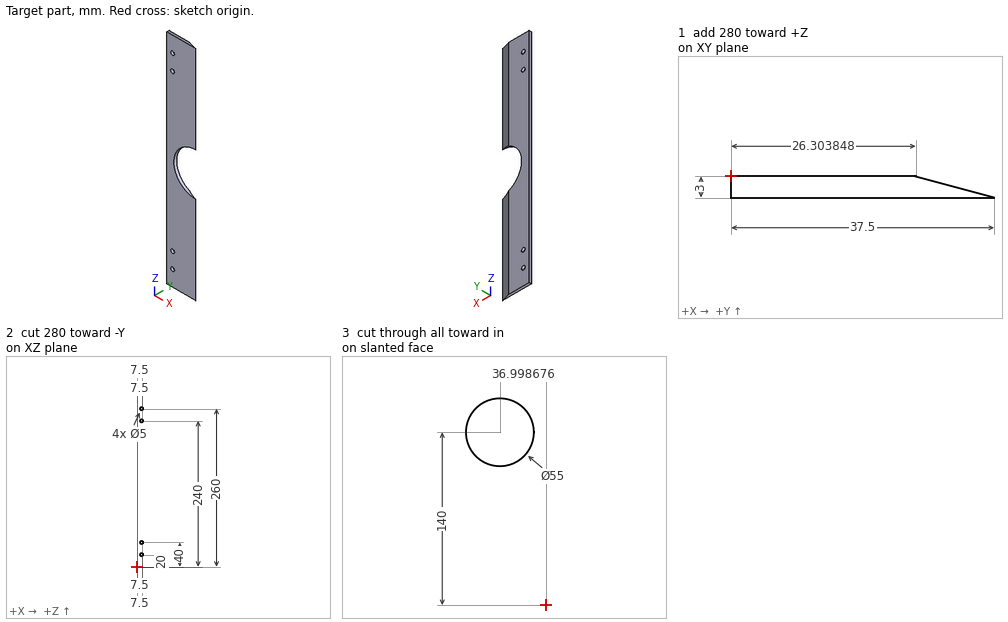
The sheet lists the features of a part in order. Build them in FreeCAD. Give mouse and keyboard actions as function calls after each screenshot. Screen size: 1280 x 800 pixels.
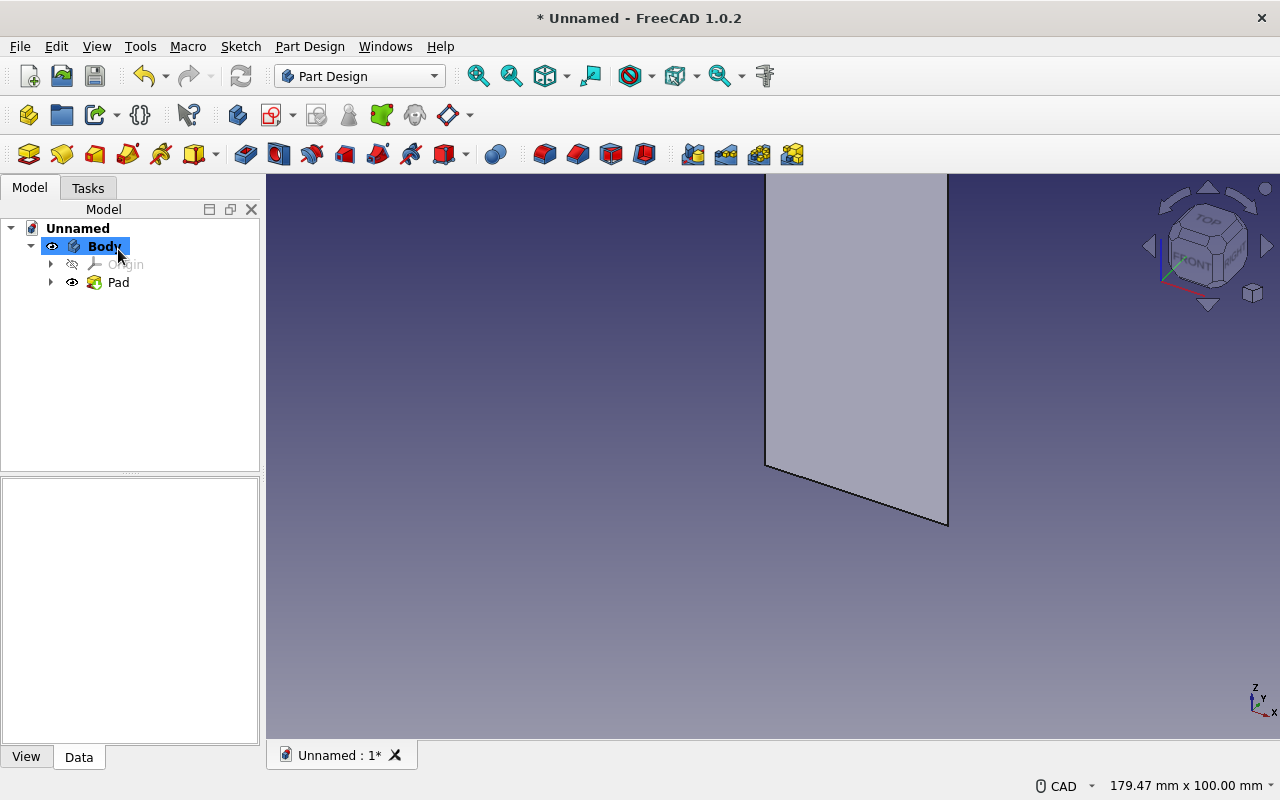
click(479, 76)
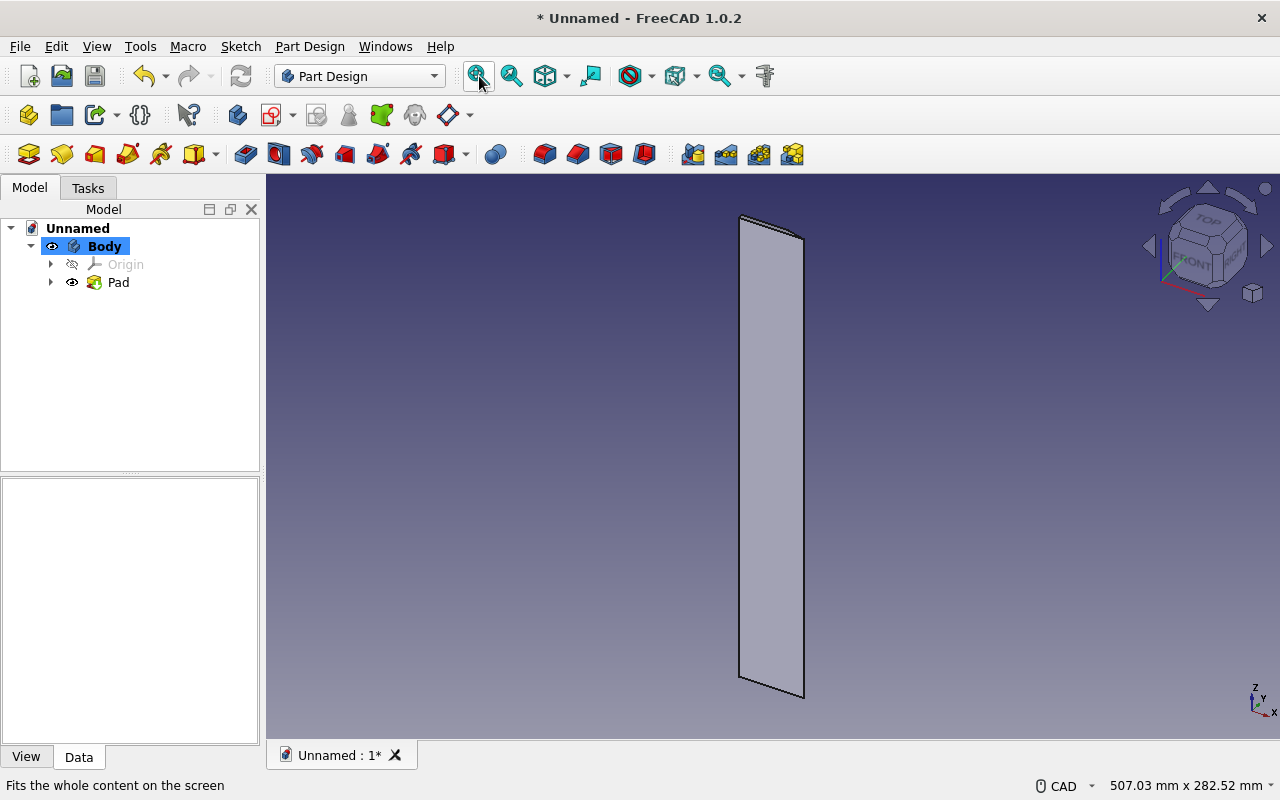
click(270, 116)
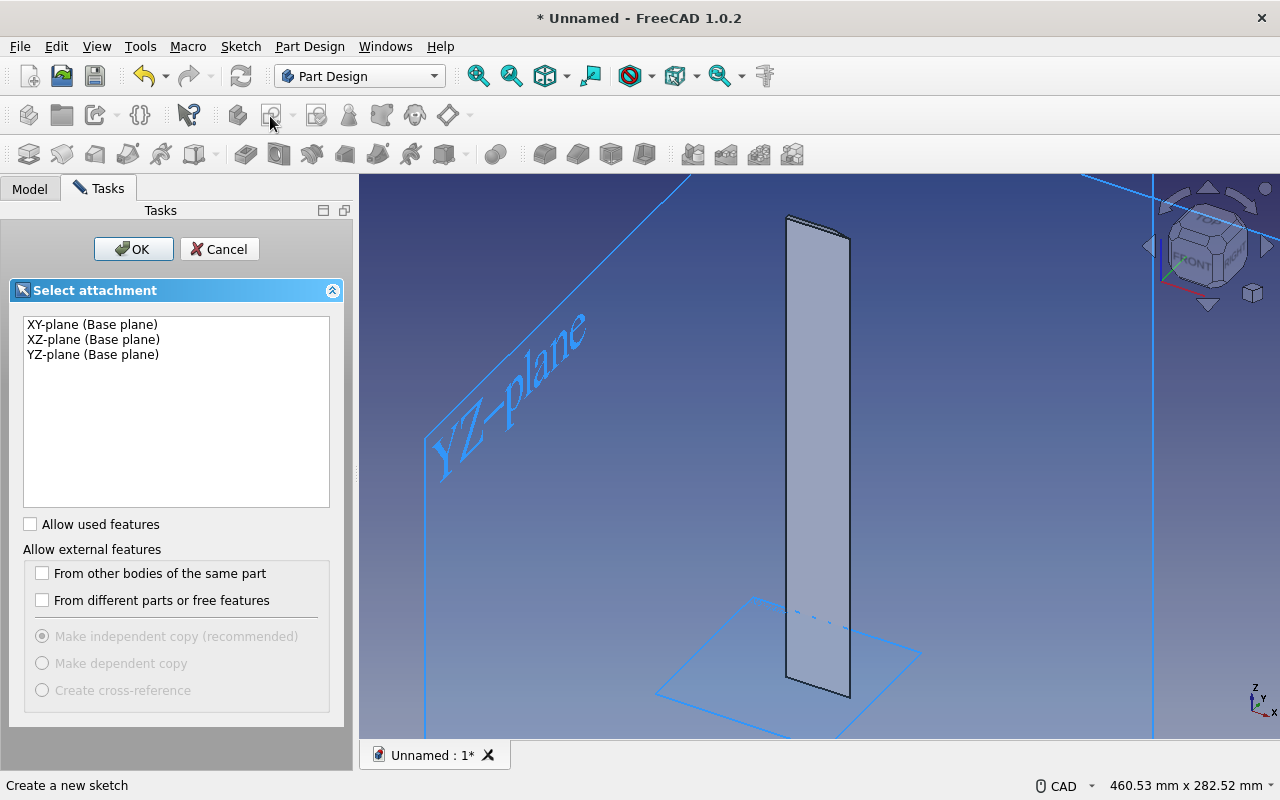
click(84, 340)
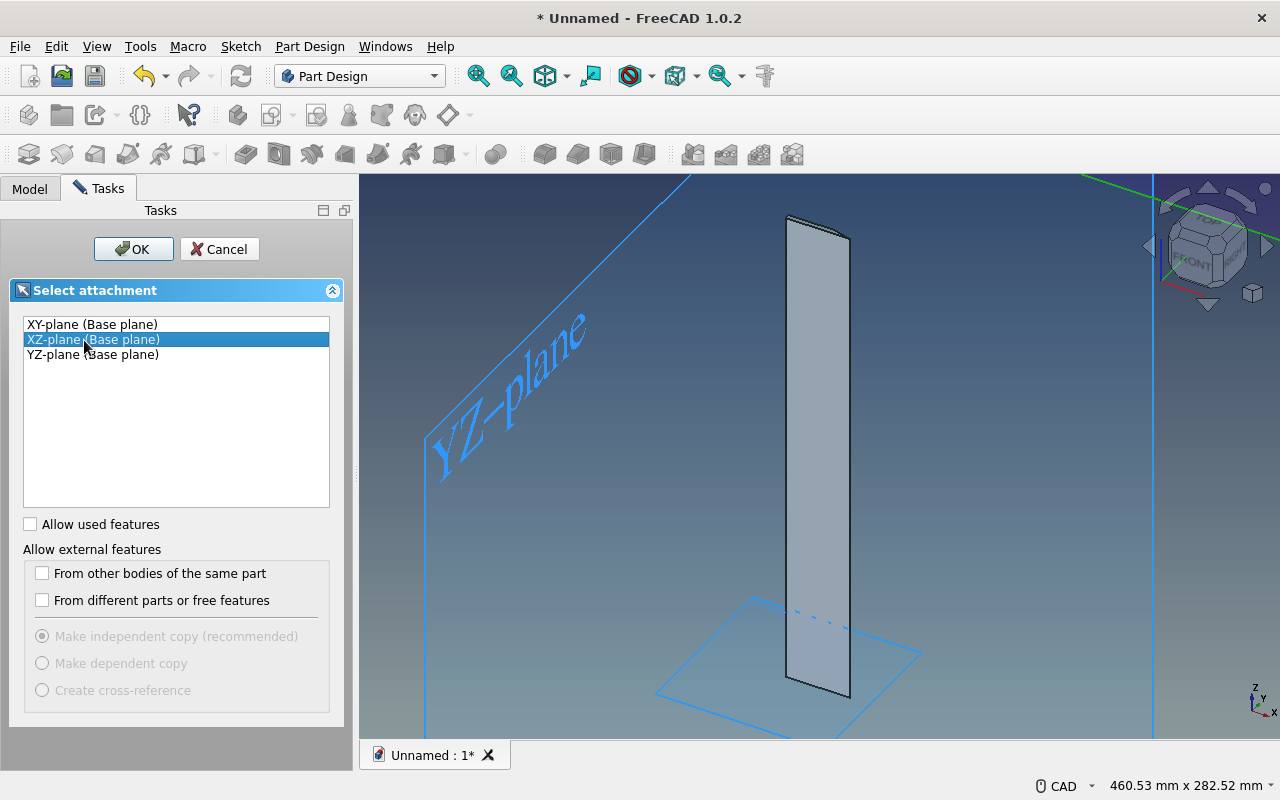
click(134, 249)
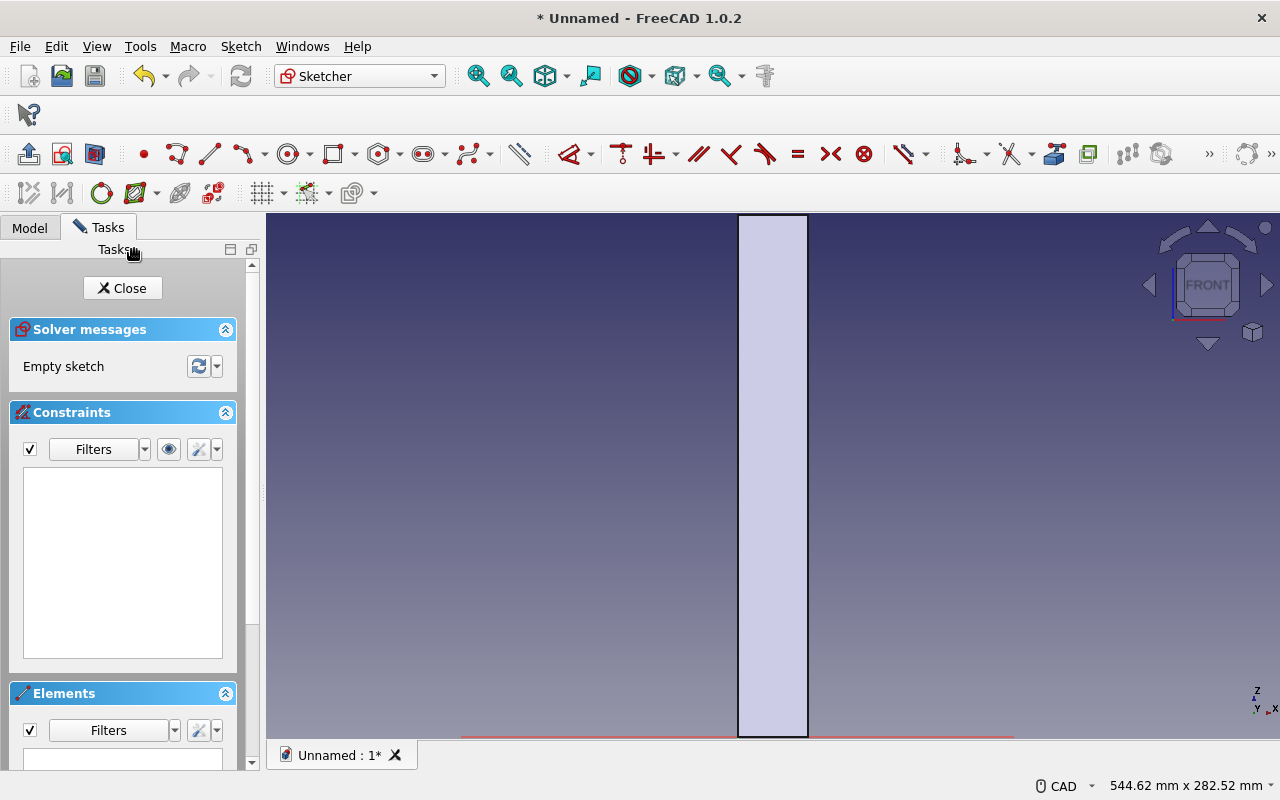
click(95, 154)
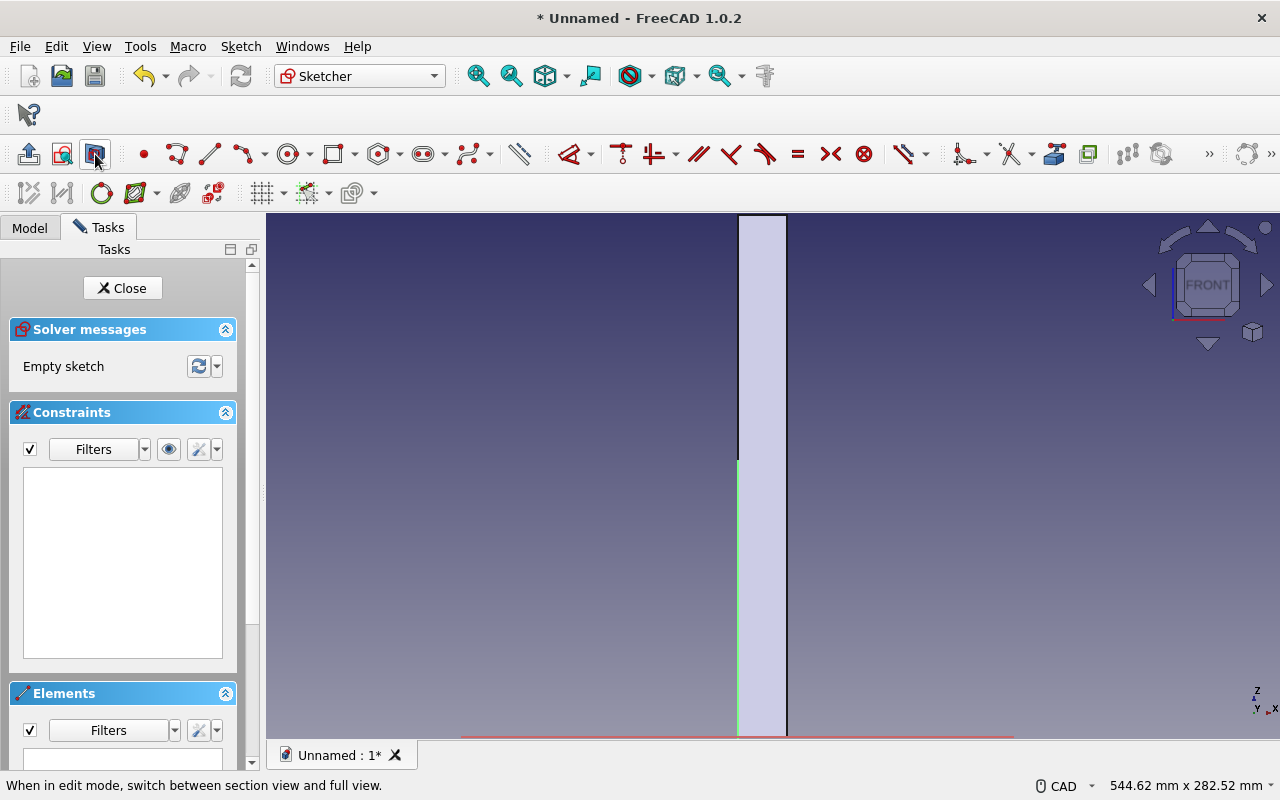
scroll(617, 443, down, 2)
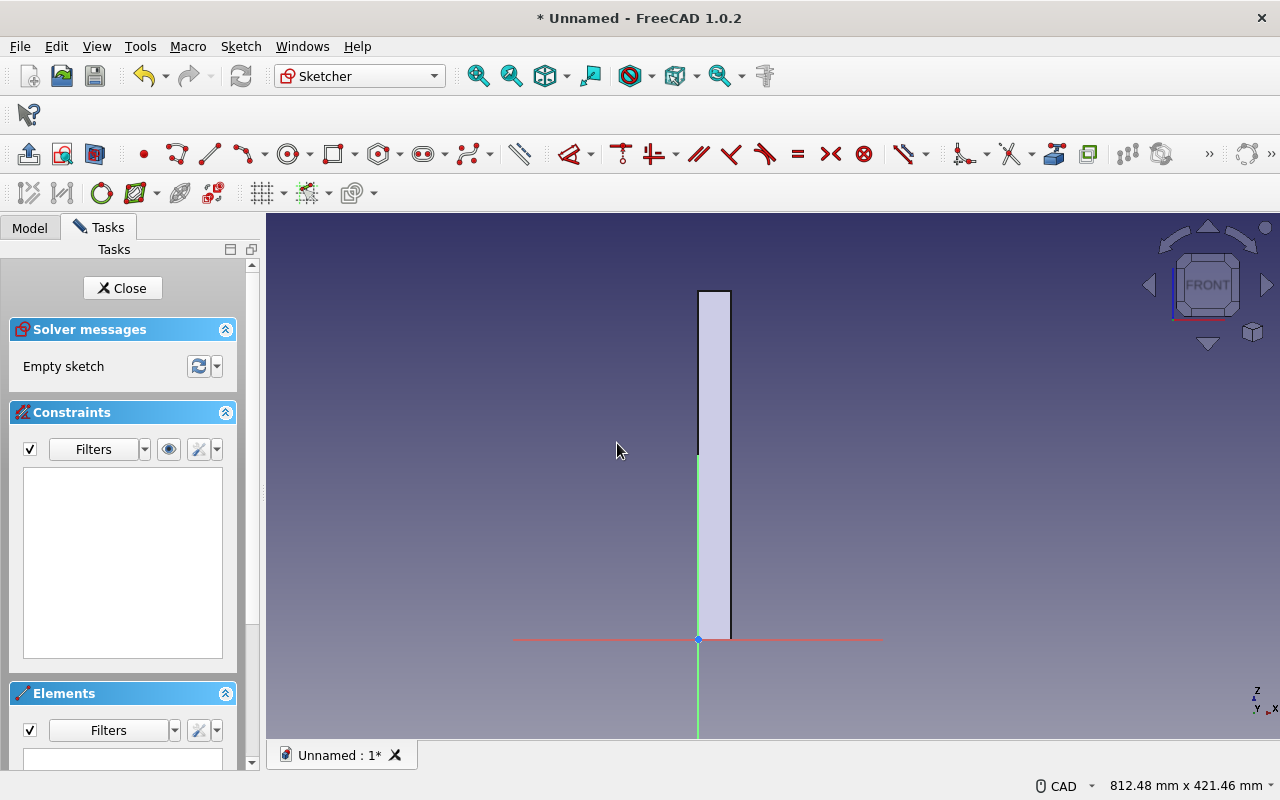
click(288, 154)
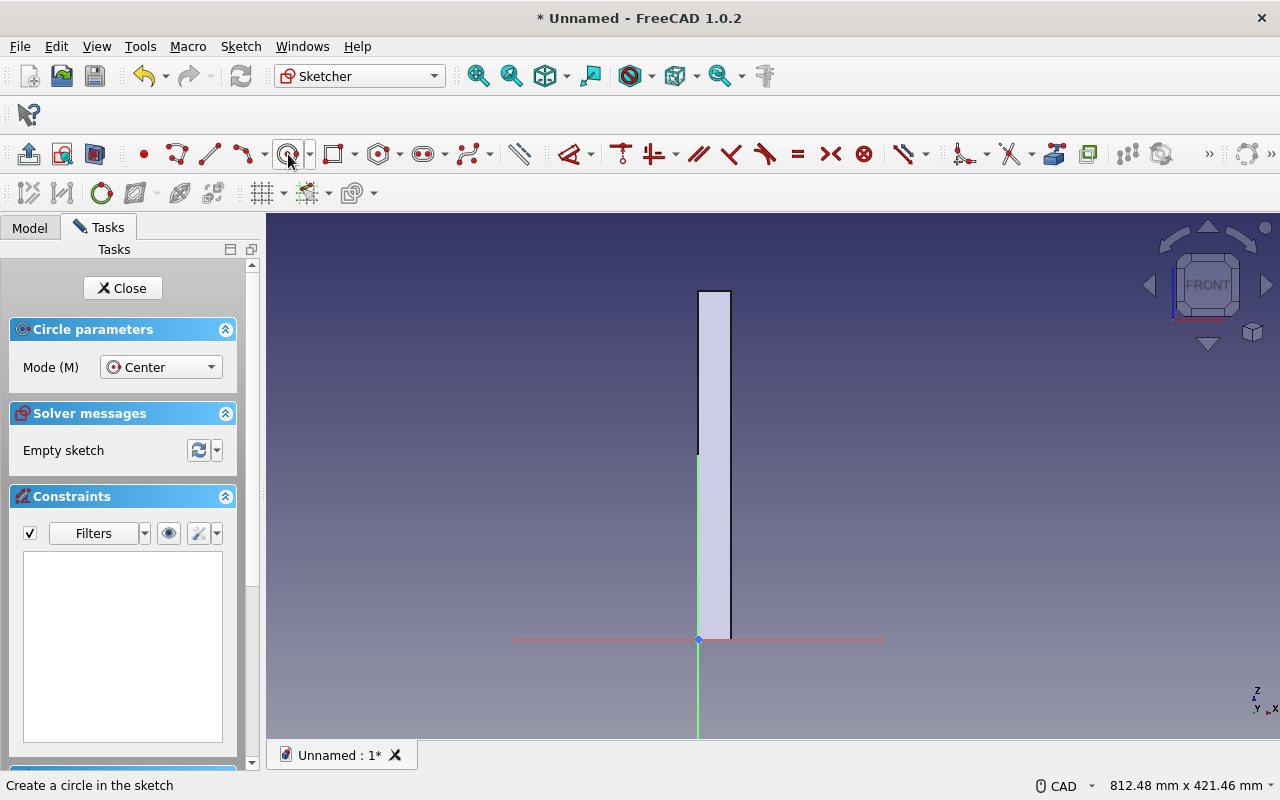
scroll(708, 316, up, 10)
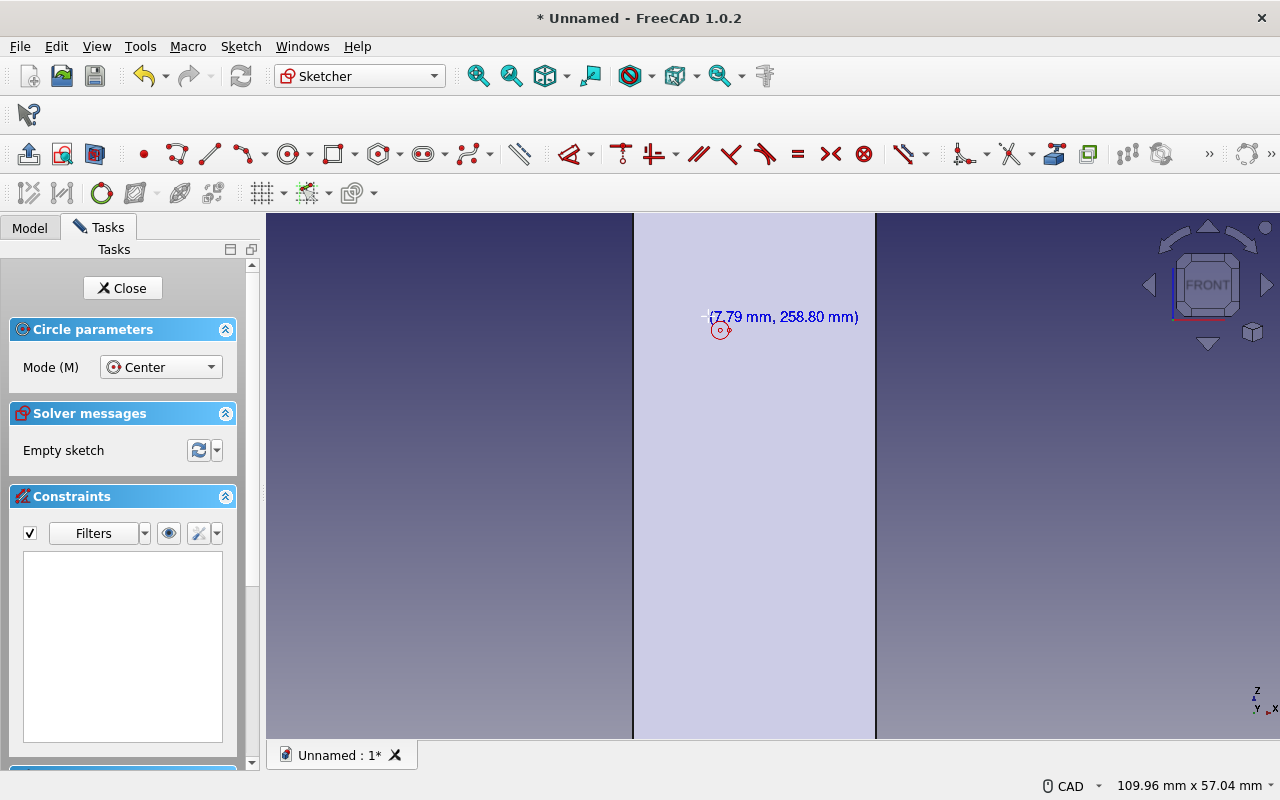
scroll(708, 316, down, 10)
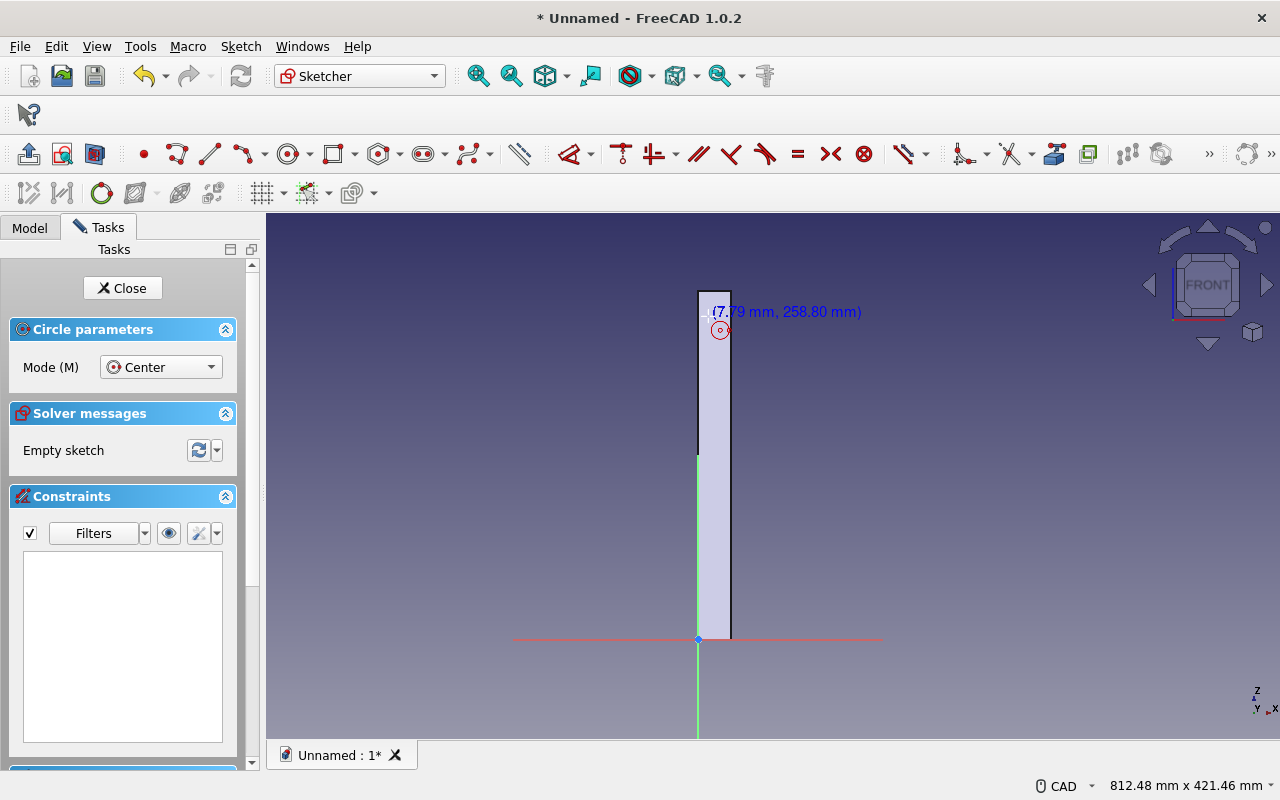
scroll(708, 316, up, 3)